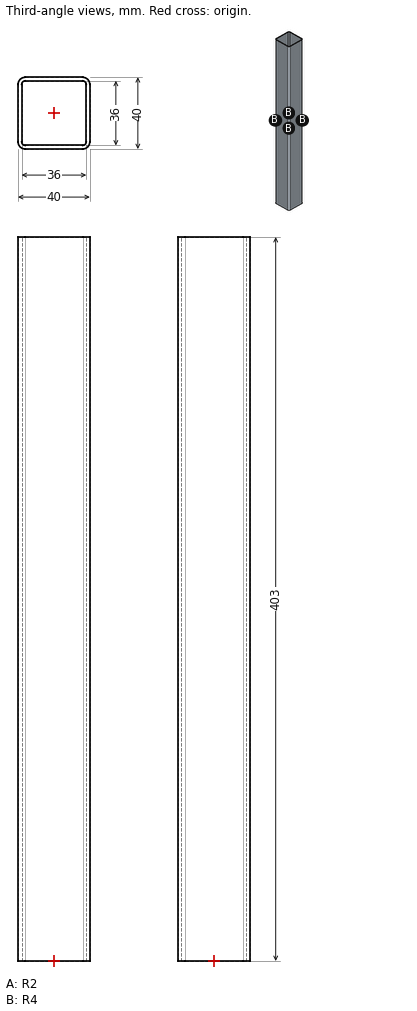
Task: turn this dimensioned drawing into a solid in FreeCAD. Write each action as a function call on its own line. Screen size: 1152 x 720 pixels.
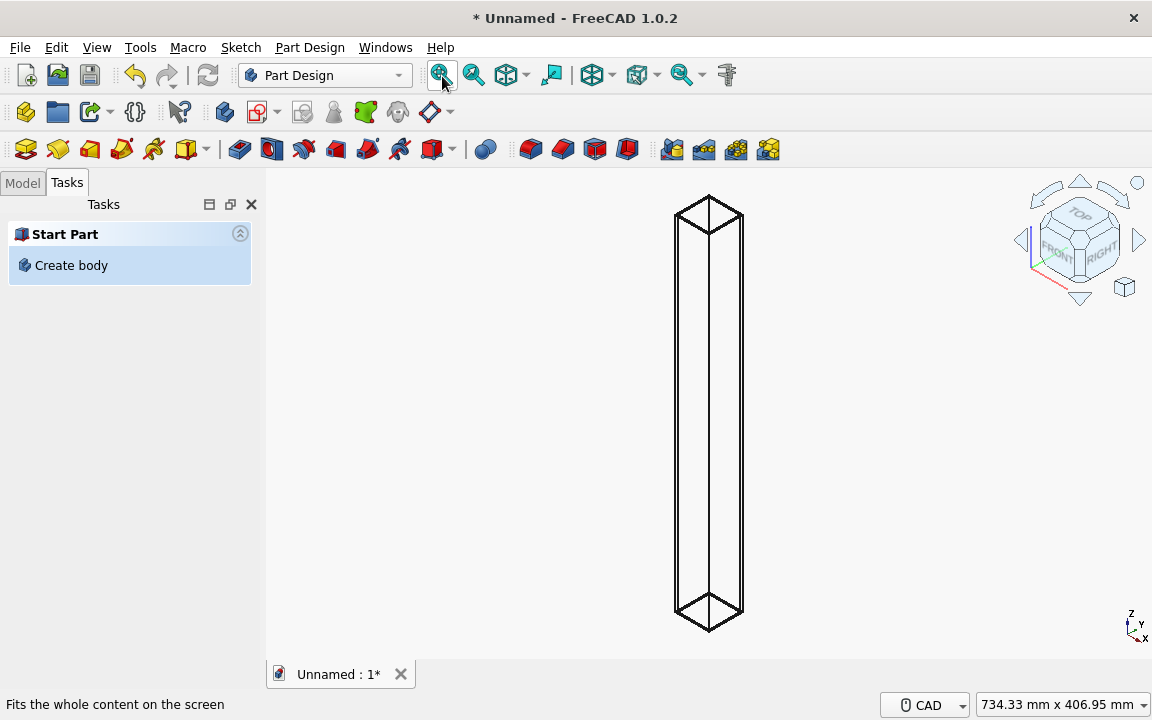
click(678, 412)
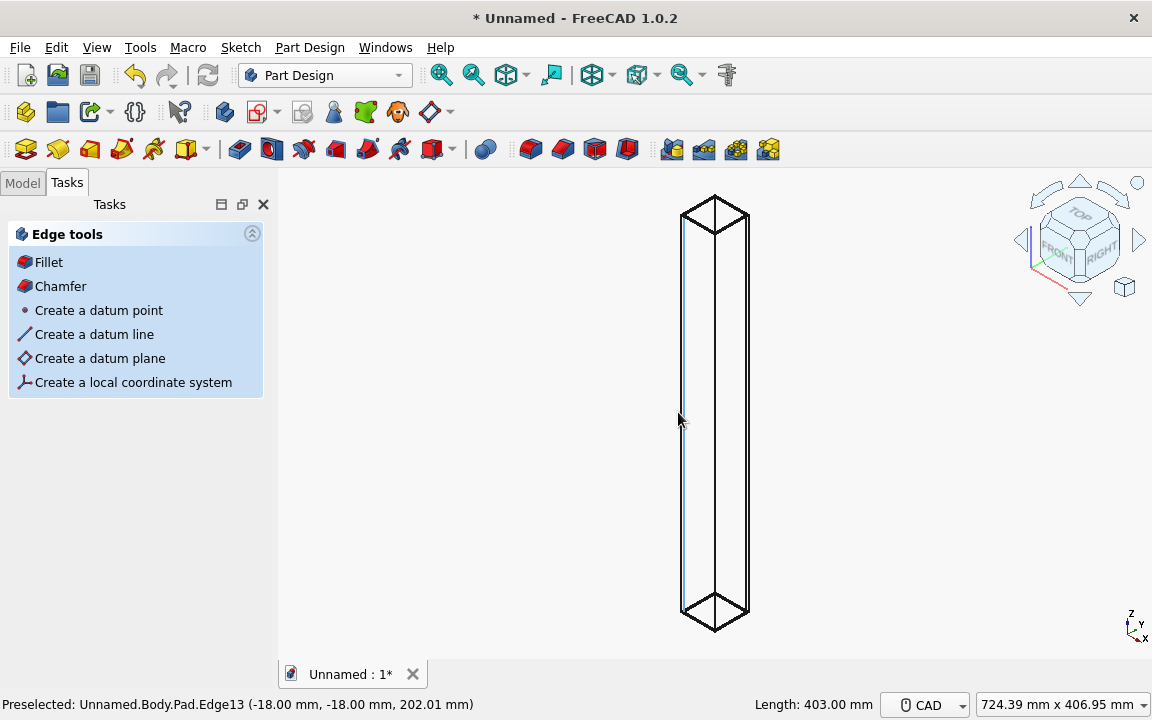
scroll(715, 430, up, 6)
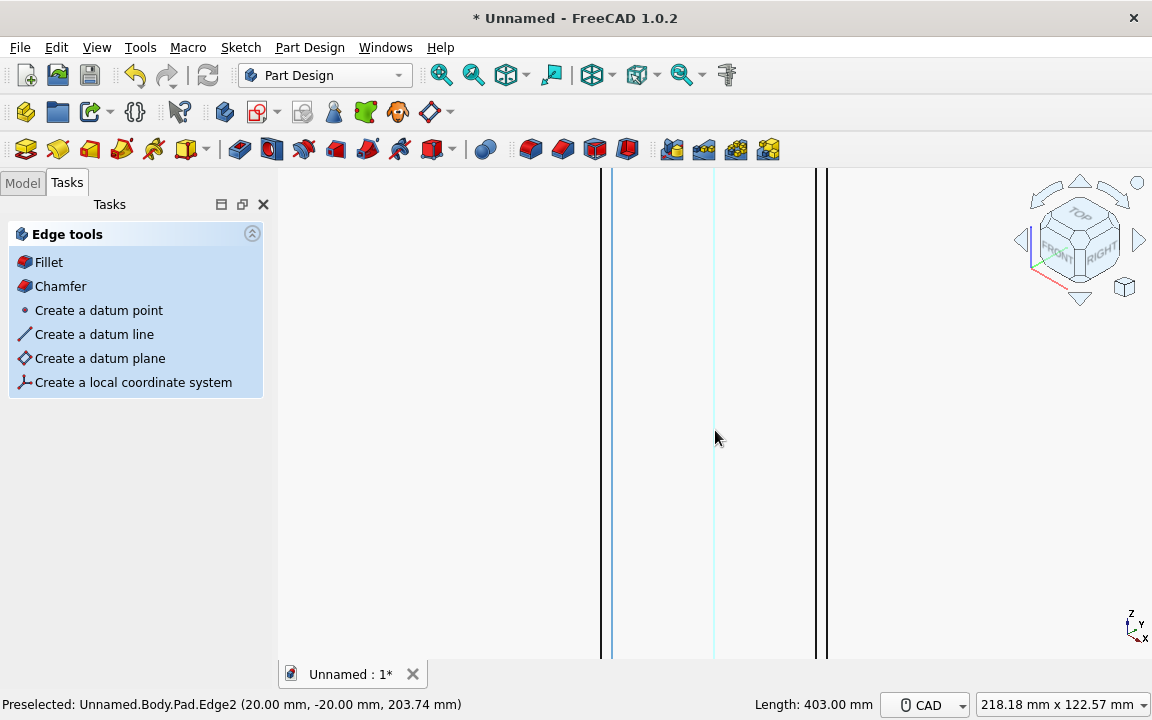
click(816, 373, ctrl)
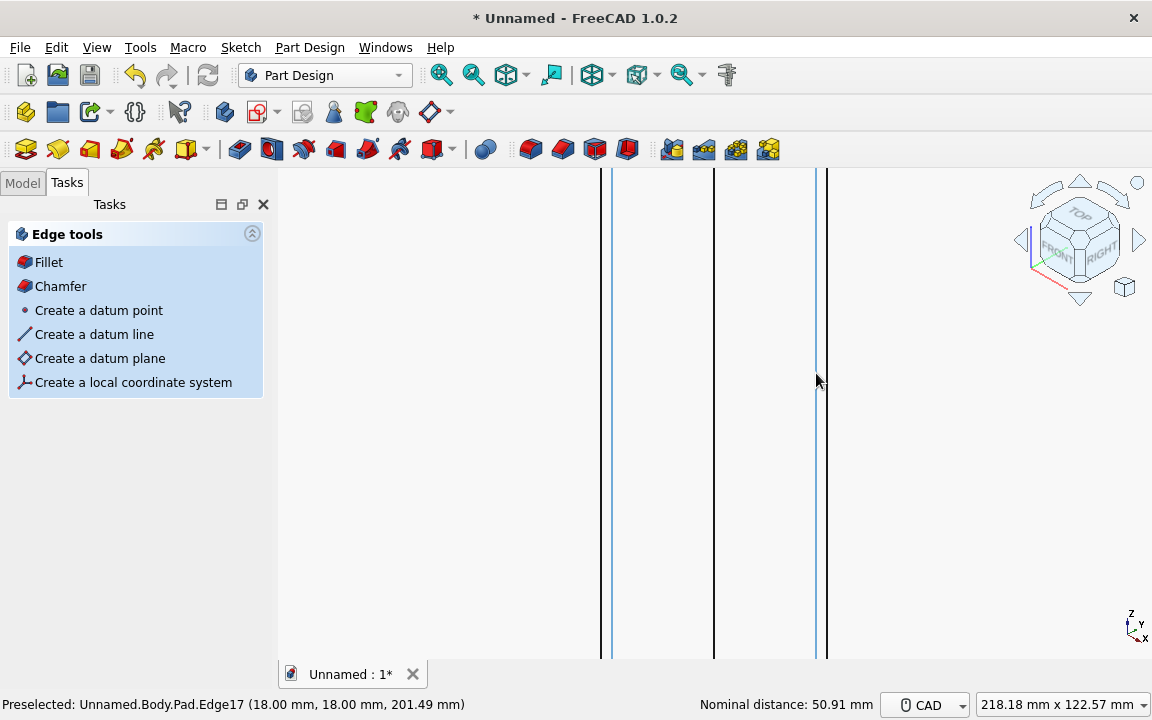
key(v)
key(f)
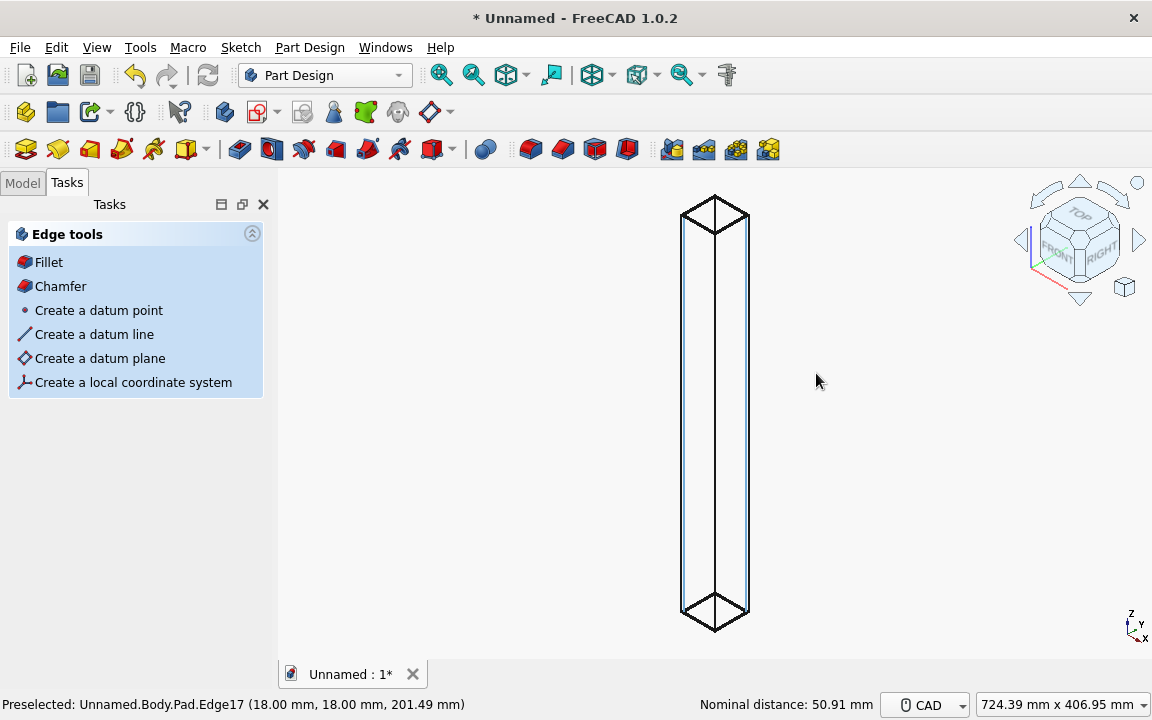
key(2)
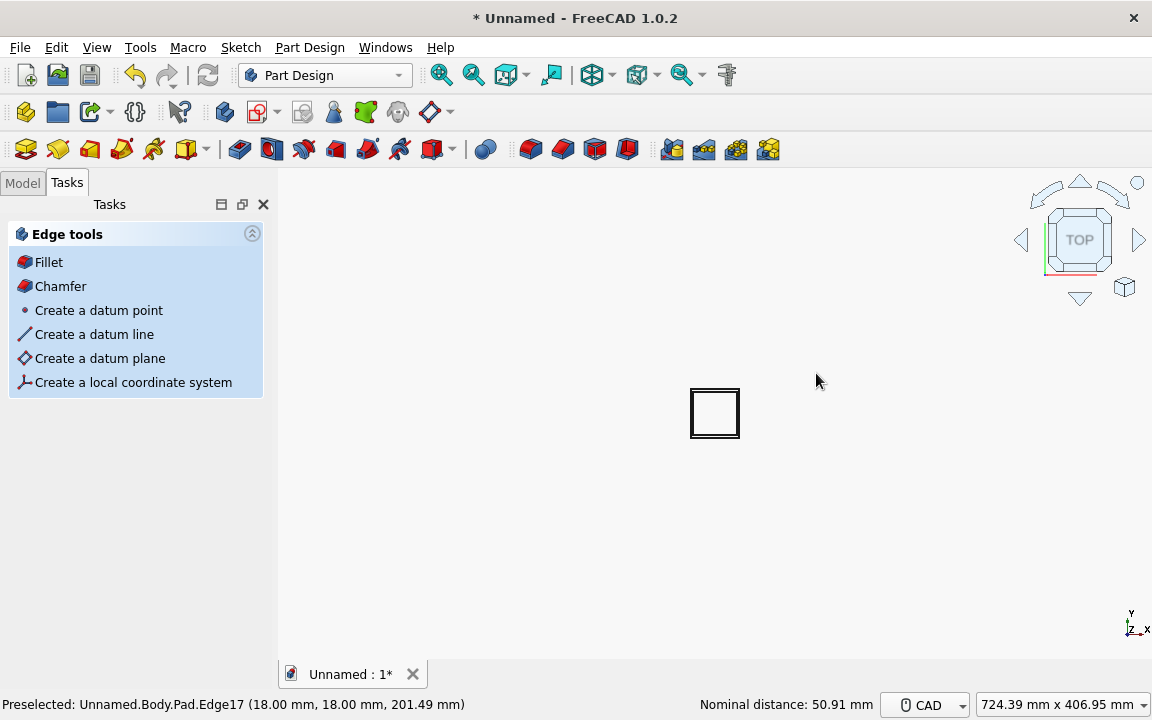
key(v)
key(f)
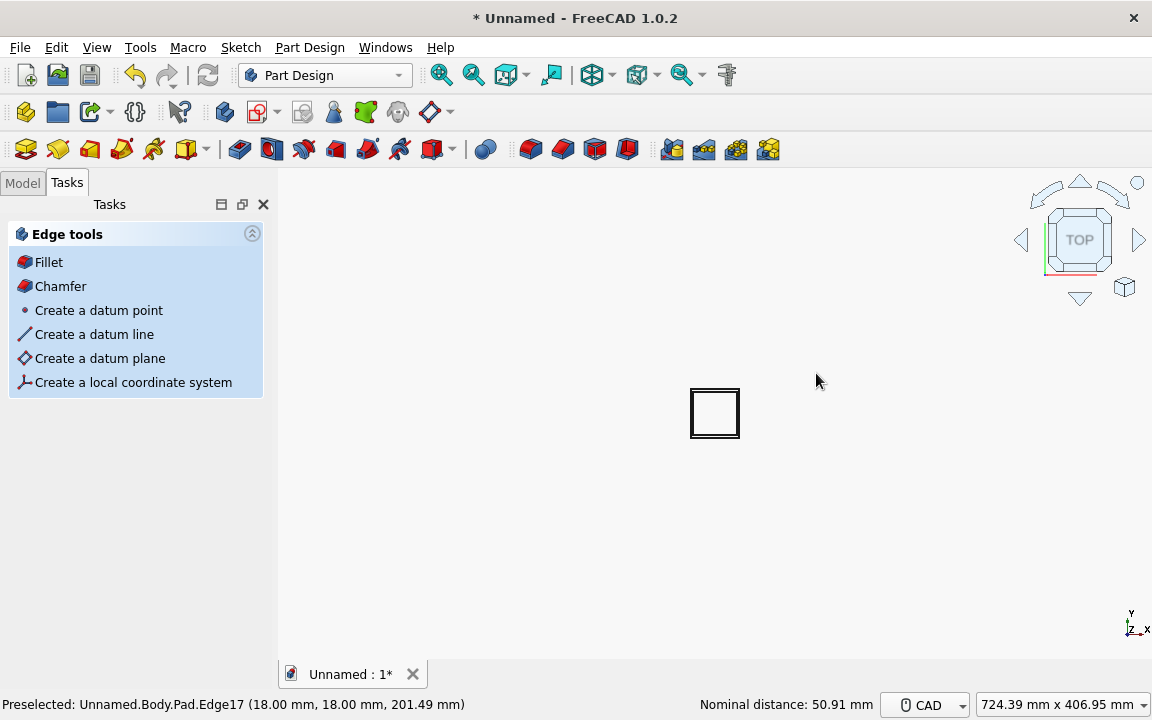
scroll(737, 434, up, 6)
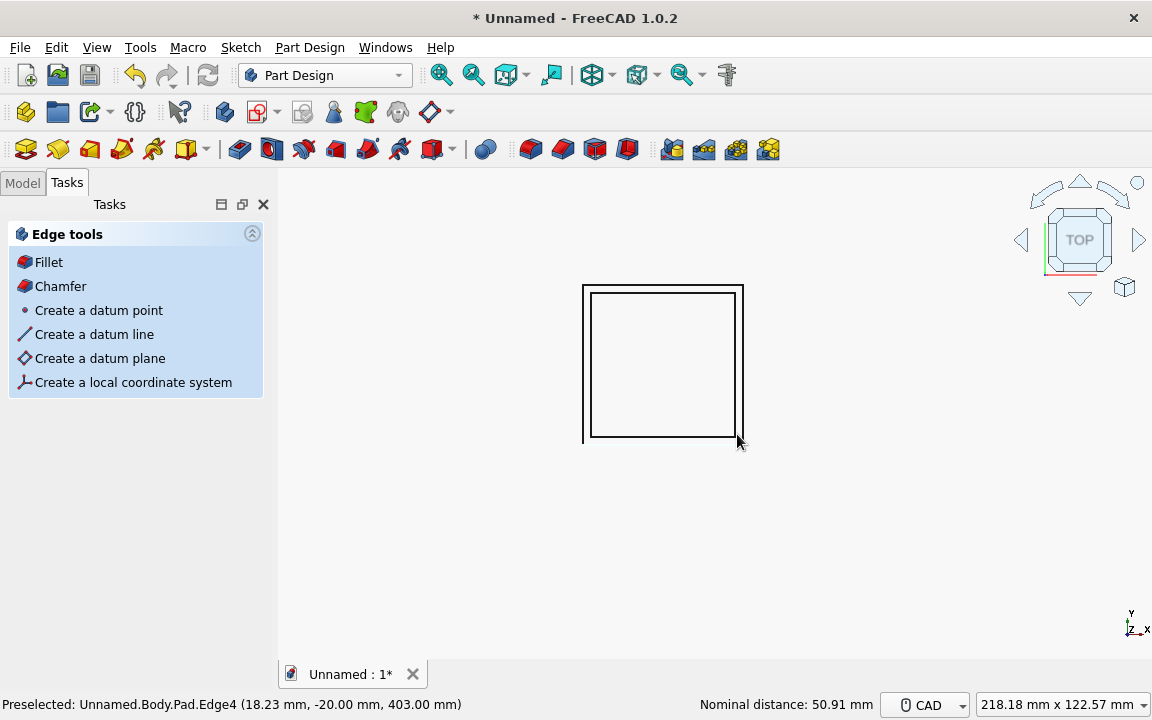
key(v)
key(f)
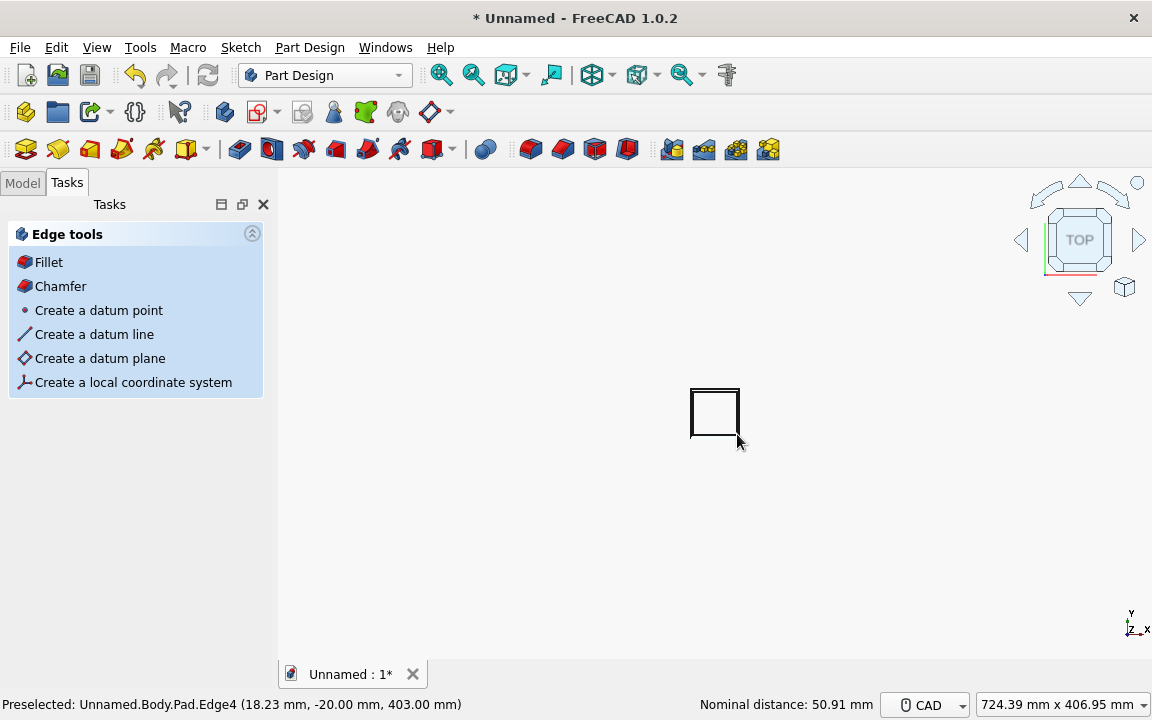
key(1)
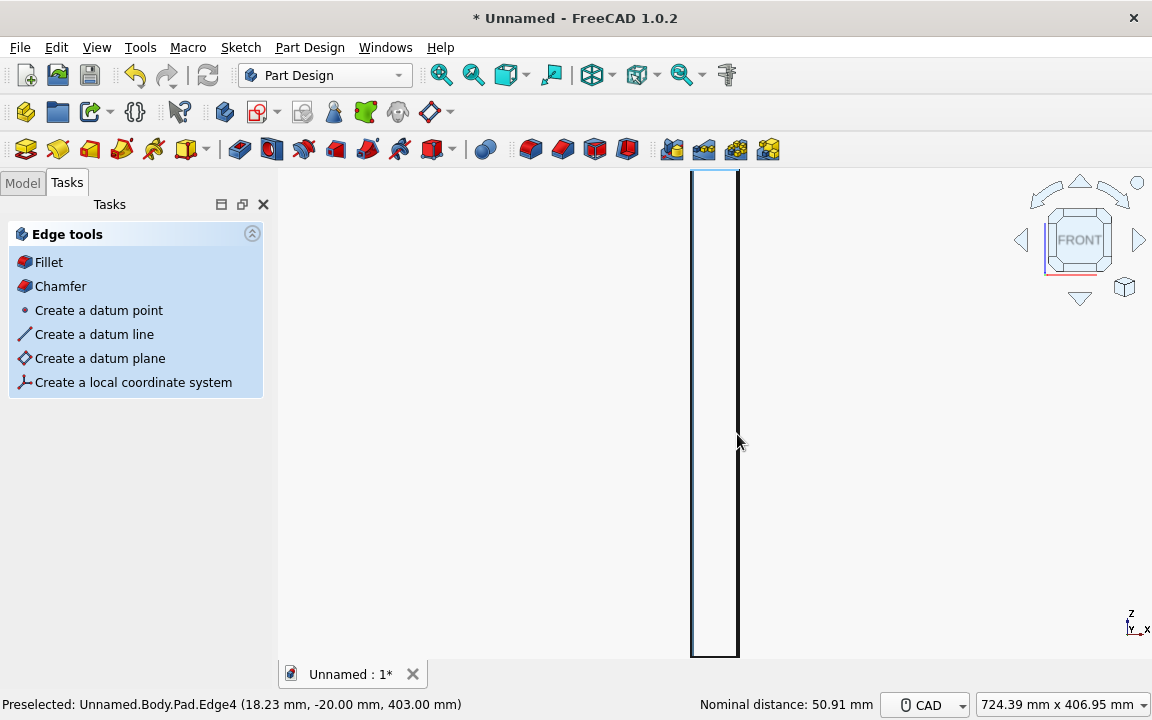
scroll(737, 412, up, 6)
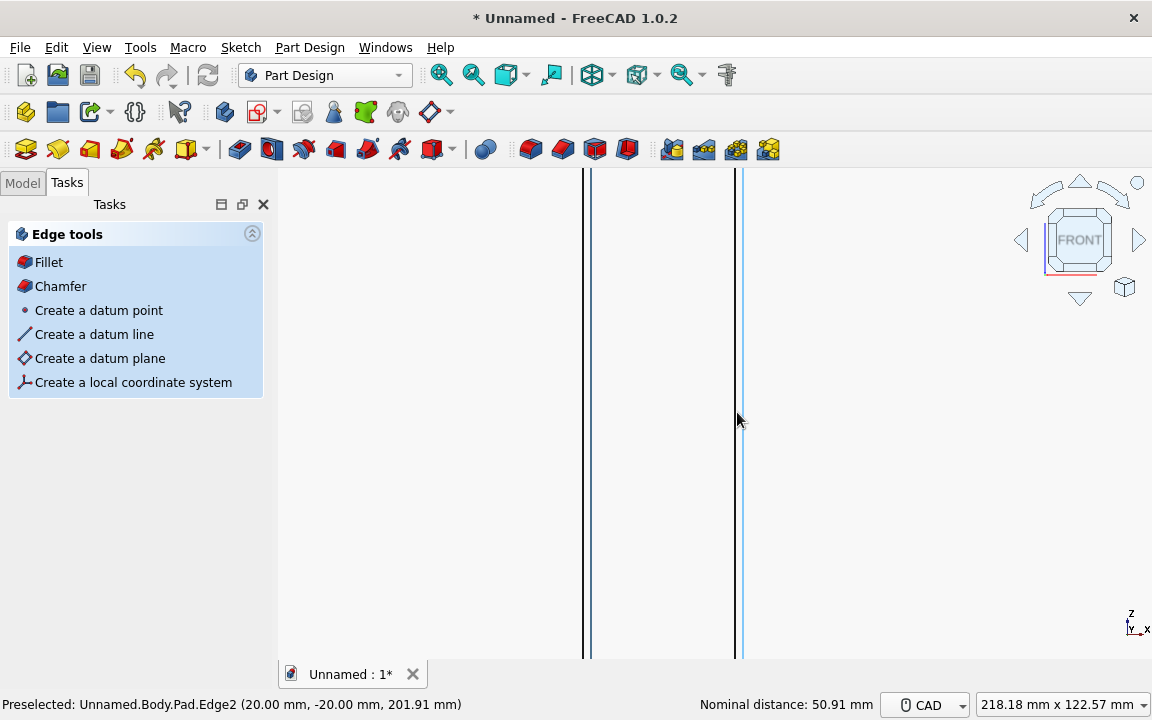
click(735, 415, ctrl)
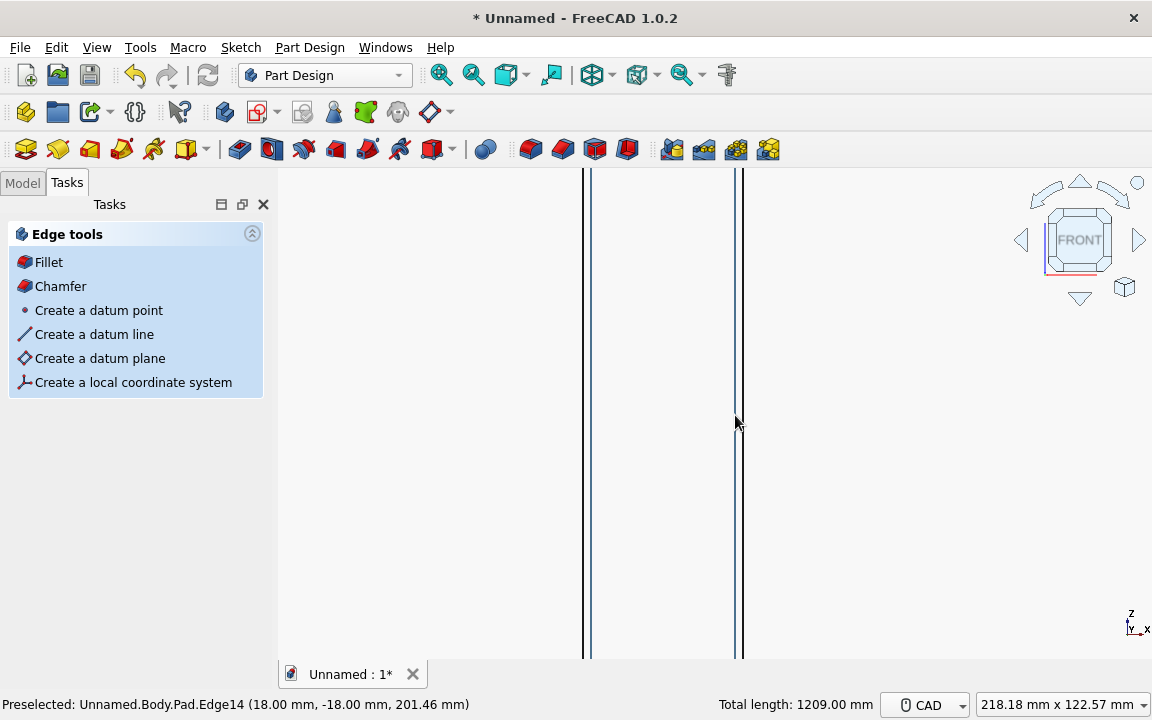
key(v)
key(f)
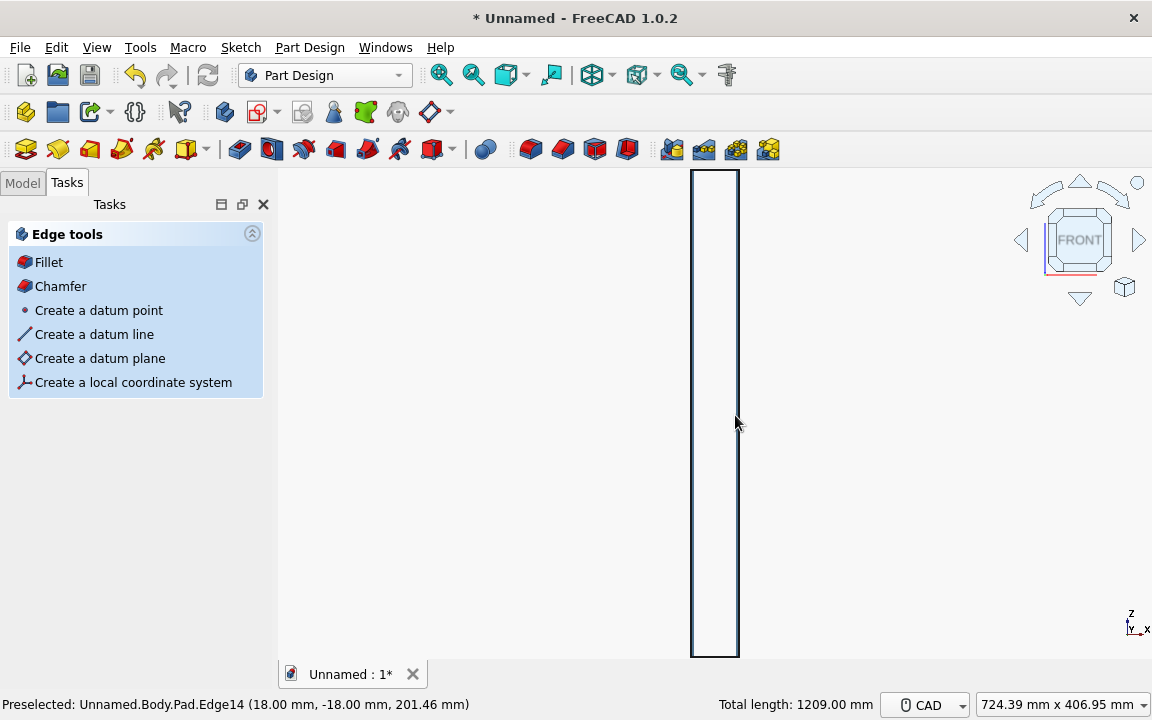
key(3)